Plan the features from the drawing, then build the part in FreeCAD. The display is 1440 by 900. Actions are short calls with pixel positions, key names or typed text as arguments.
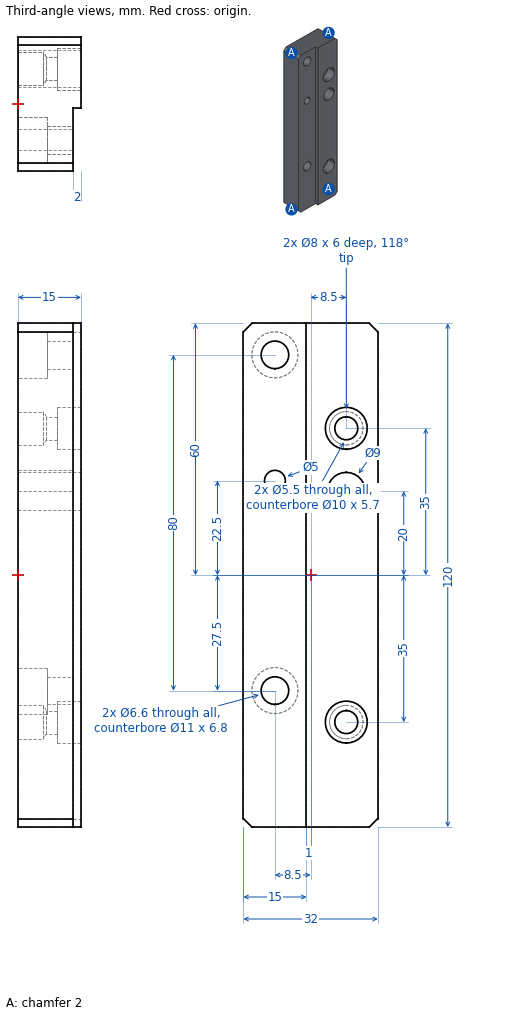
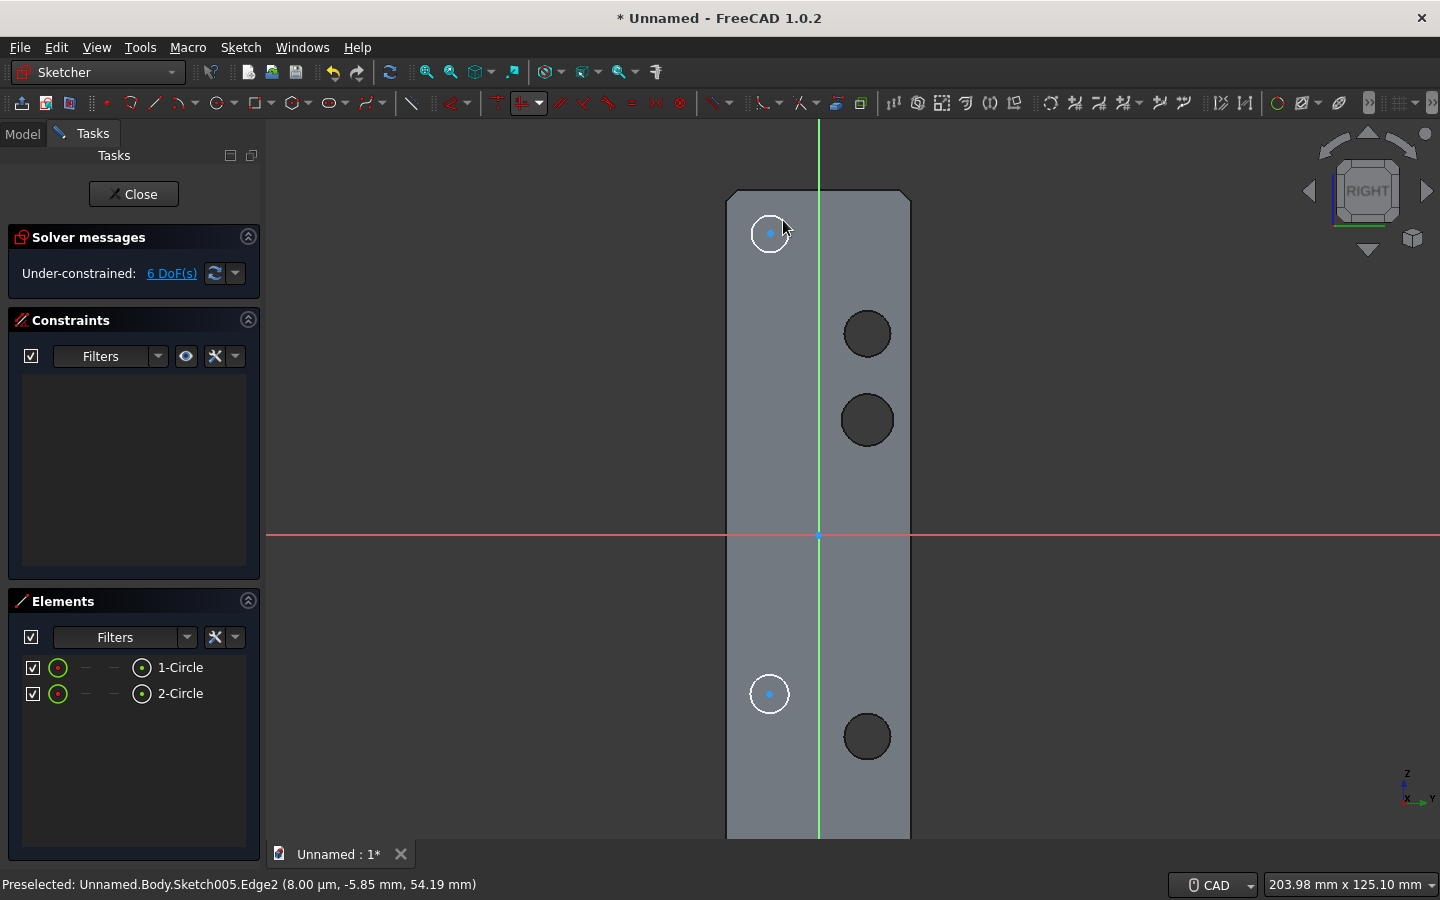
click(783, 681)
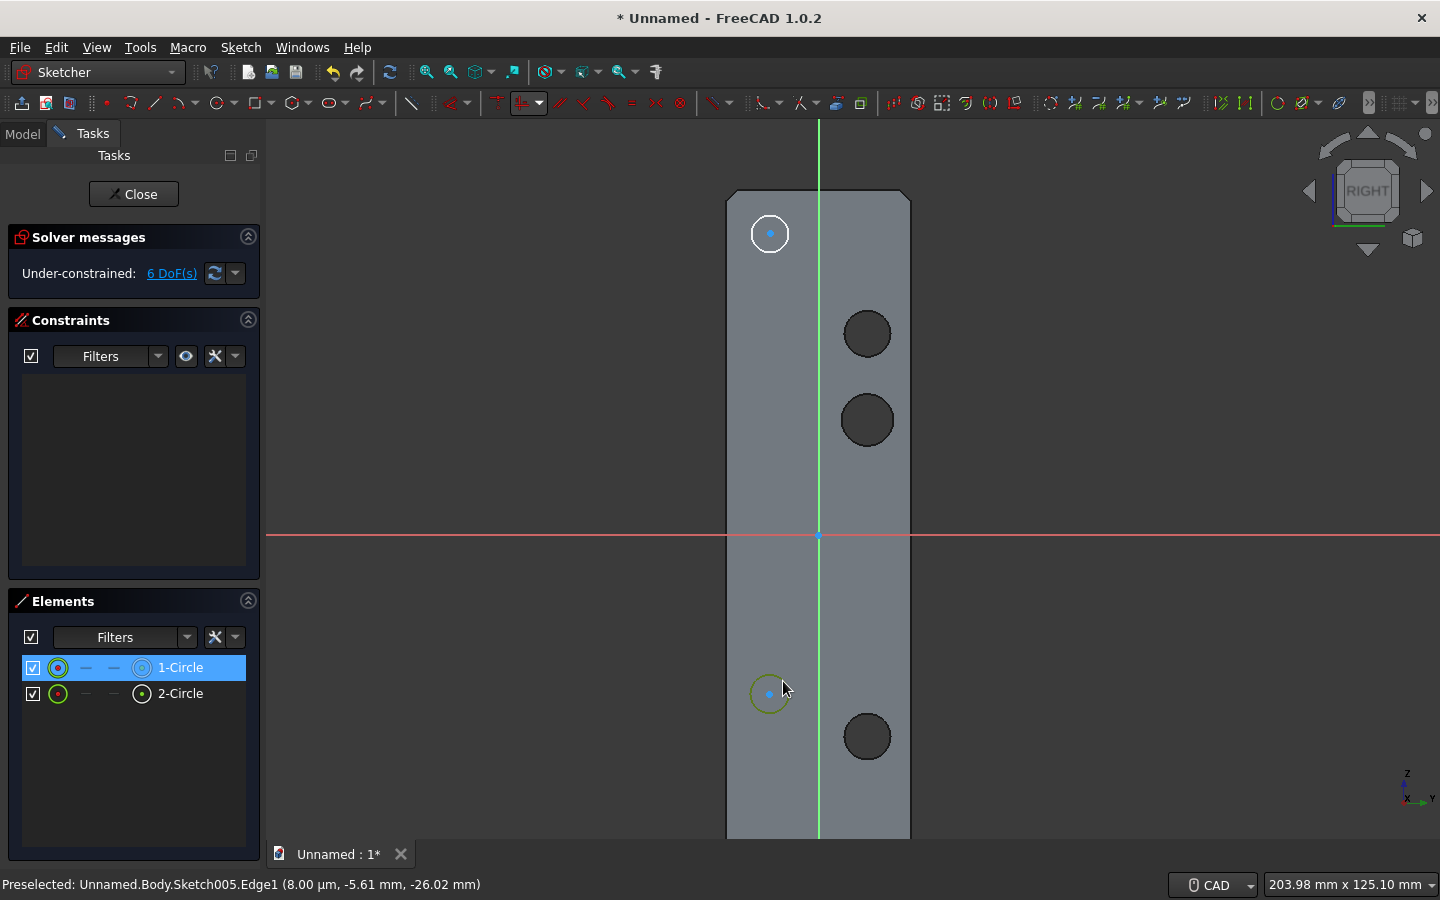
click(783, 221)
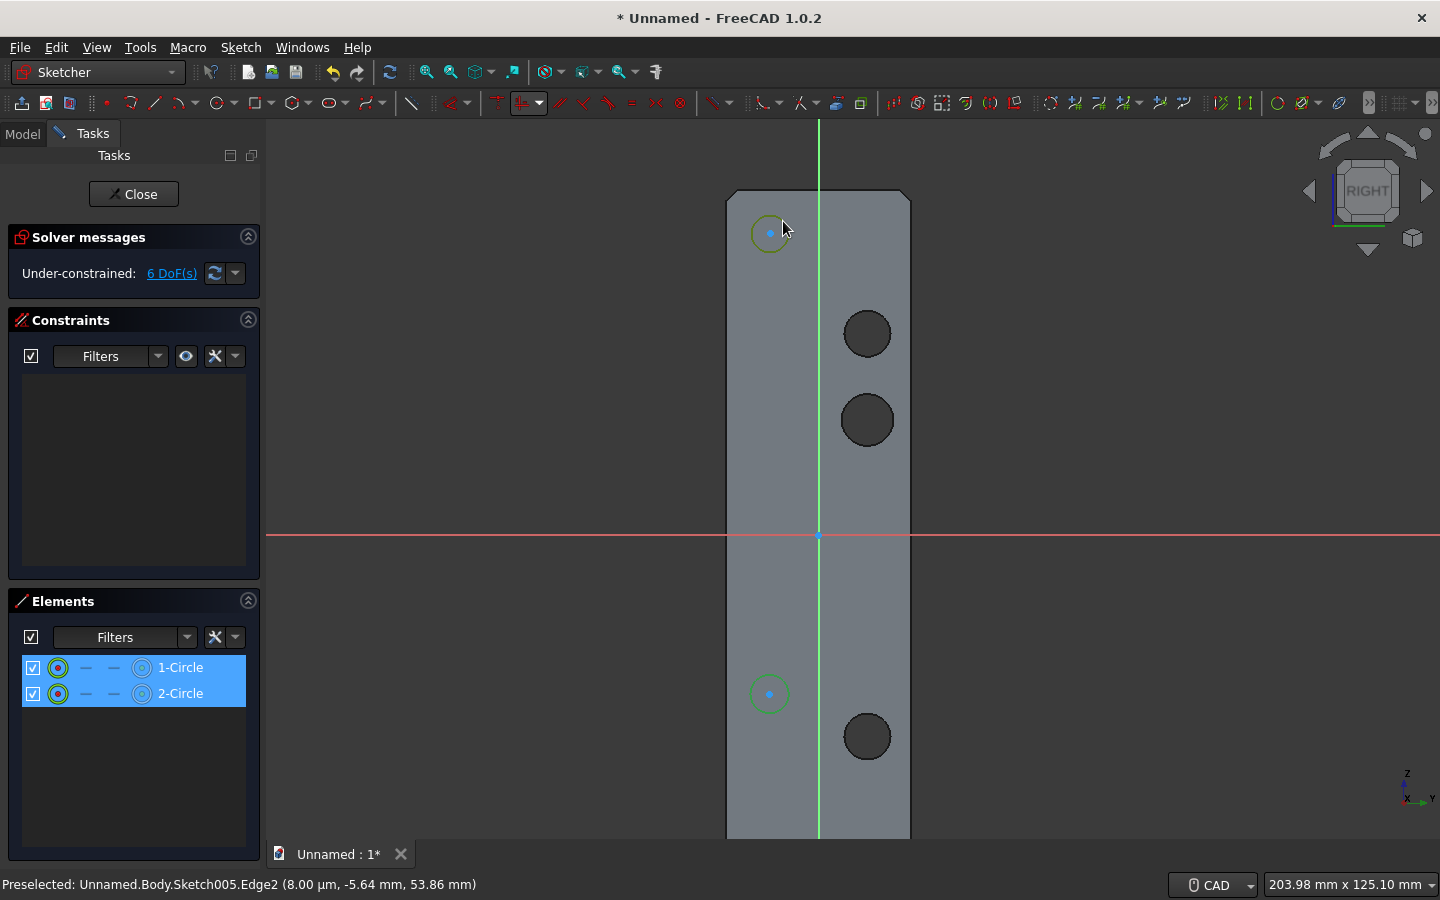
click(632, 104)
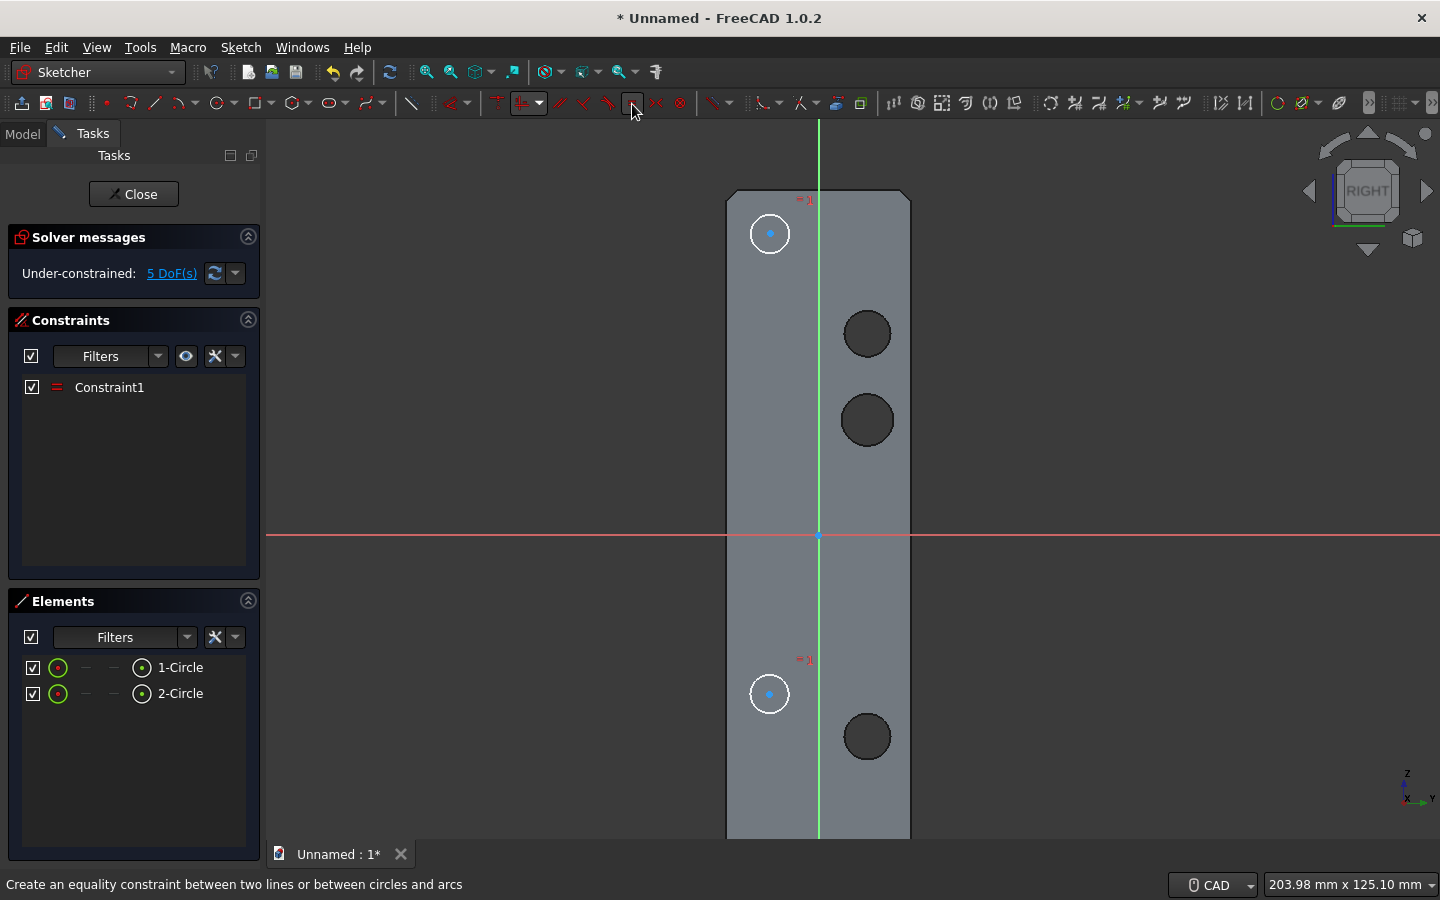
click(770, 694)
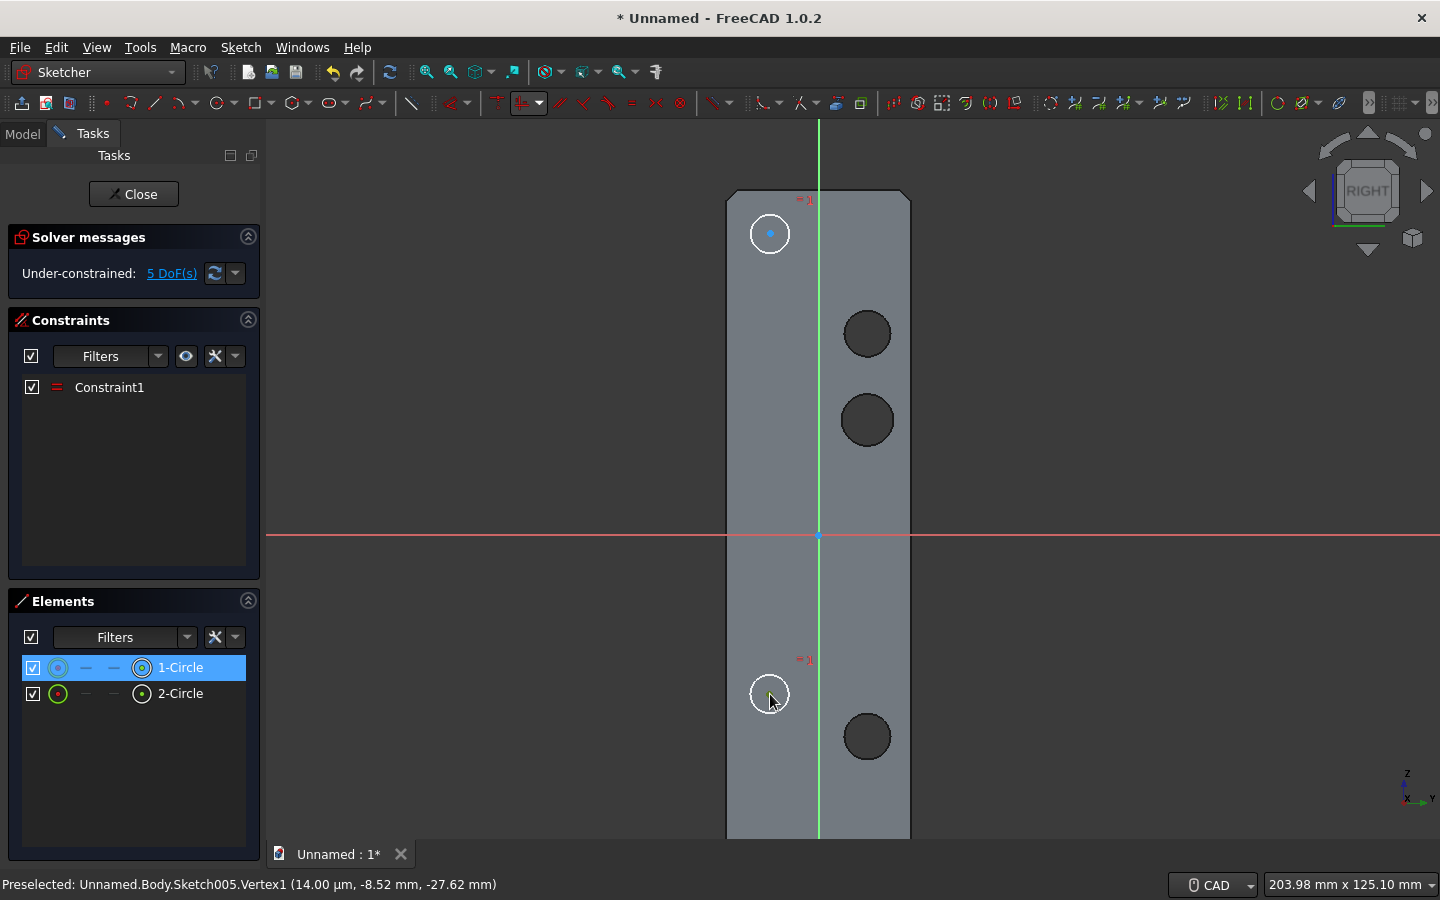
click(770, 234)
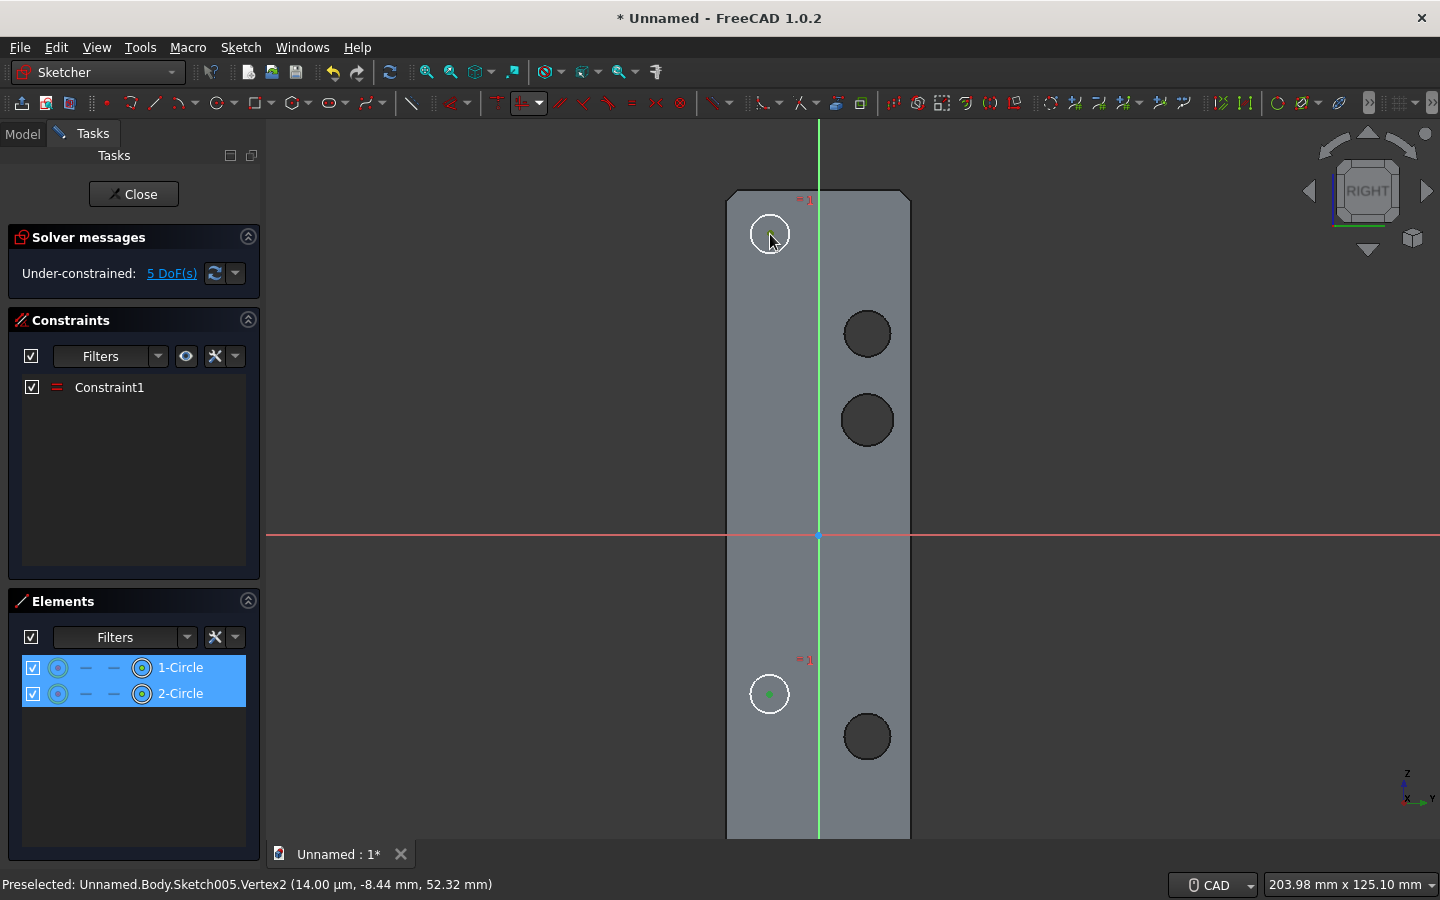
click(542, 104)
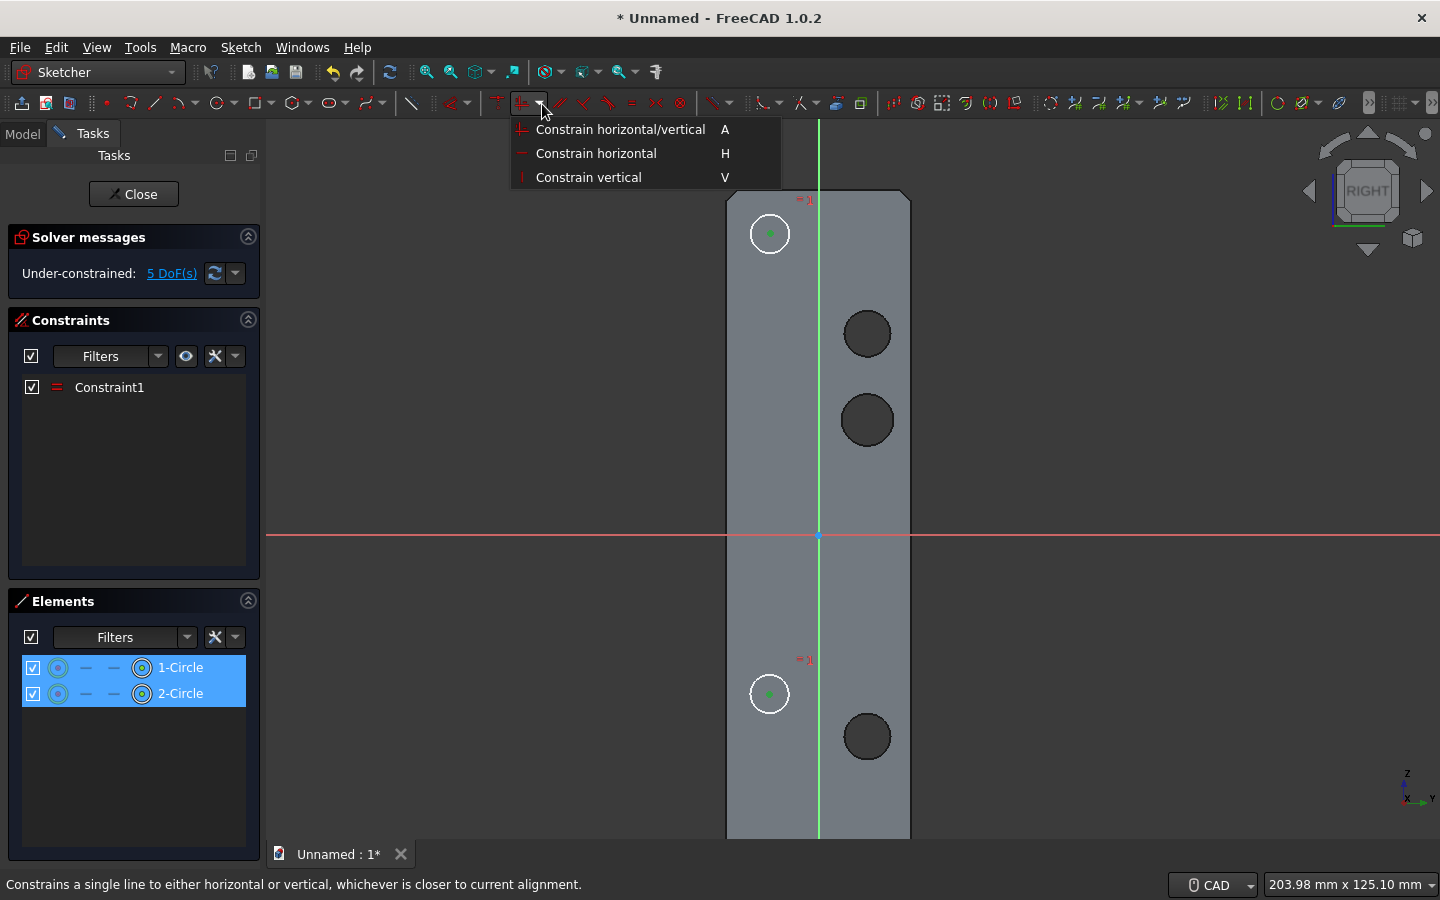
click(646, 177)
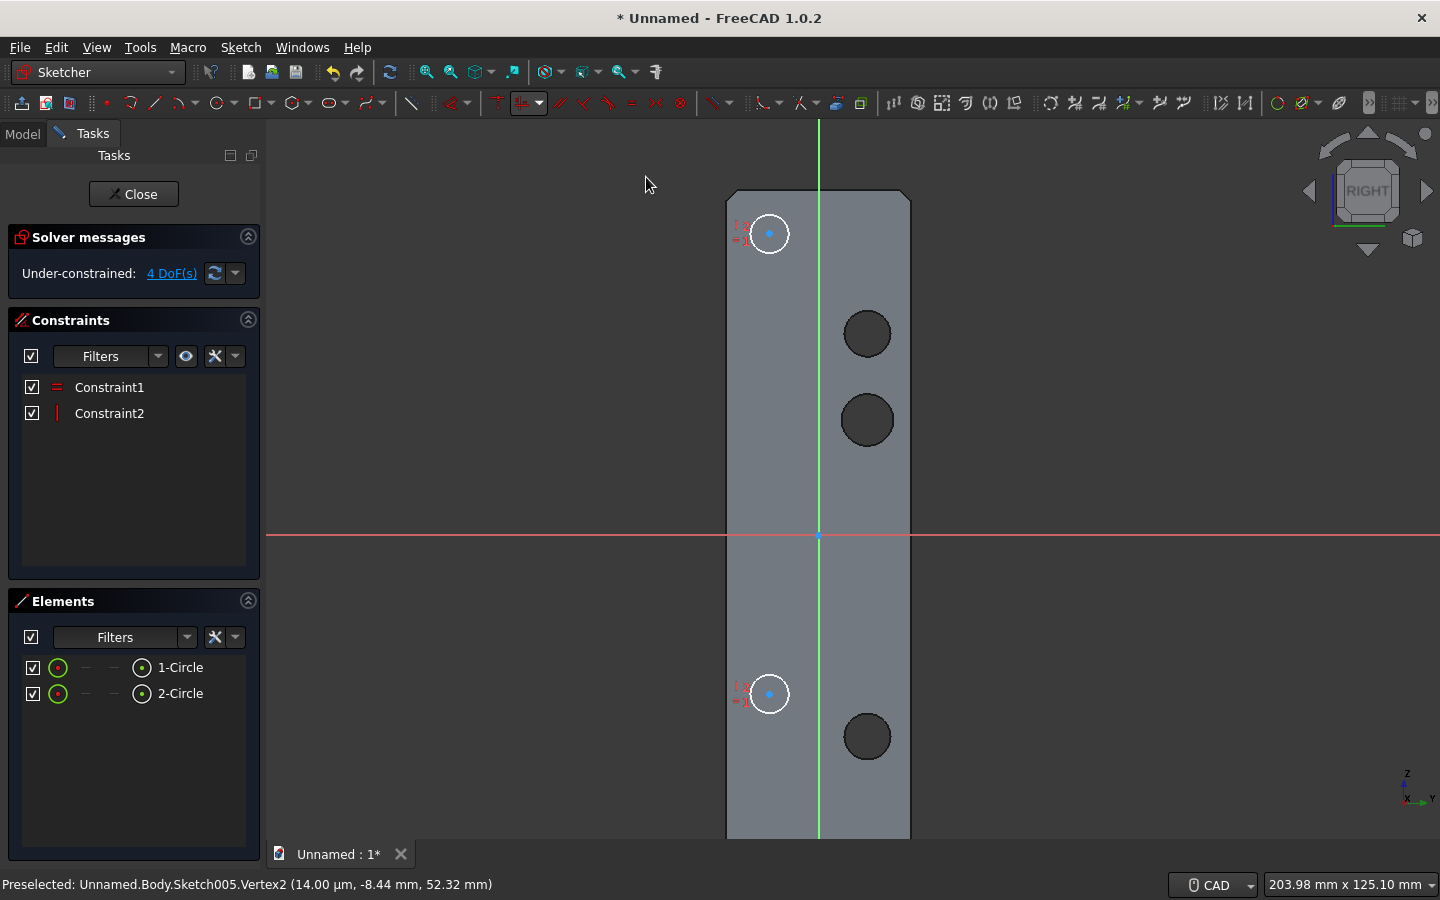
click(450, 104)